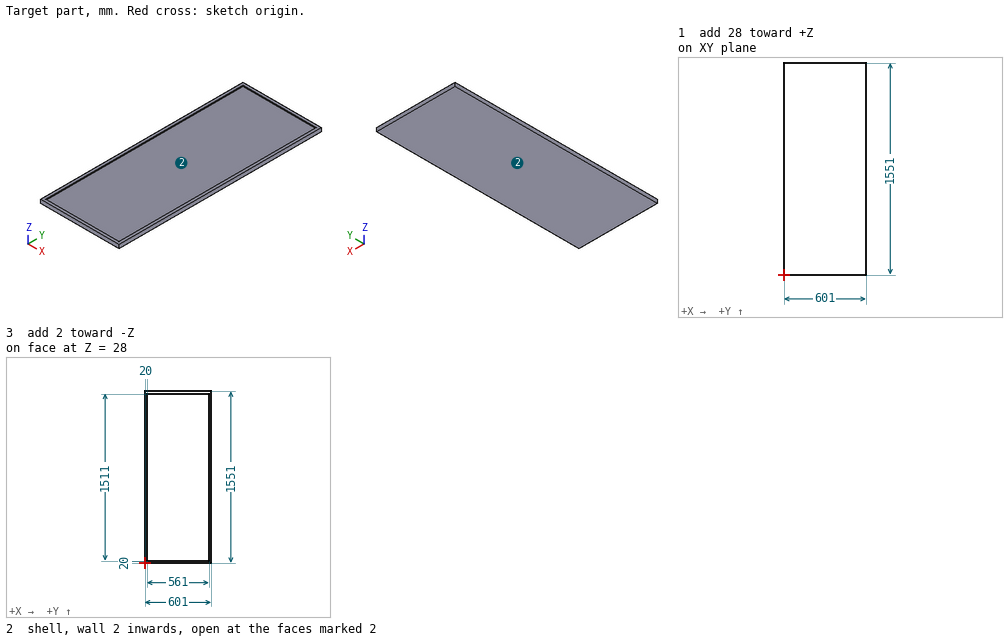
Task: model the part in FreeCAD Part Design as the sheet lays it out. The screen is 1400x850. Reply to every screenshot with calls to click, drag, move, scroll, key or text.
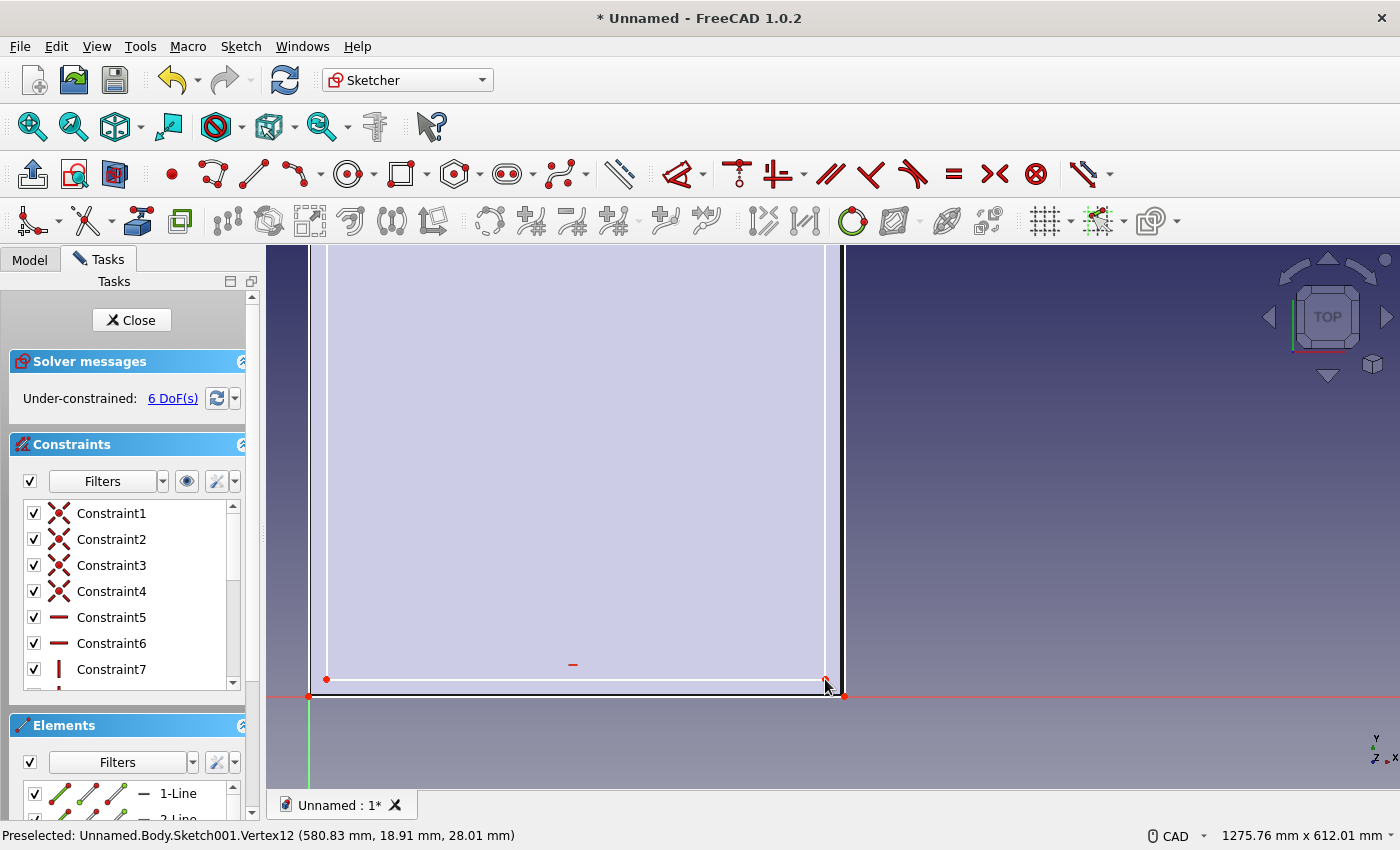
click(676, 174)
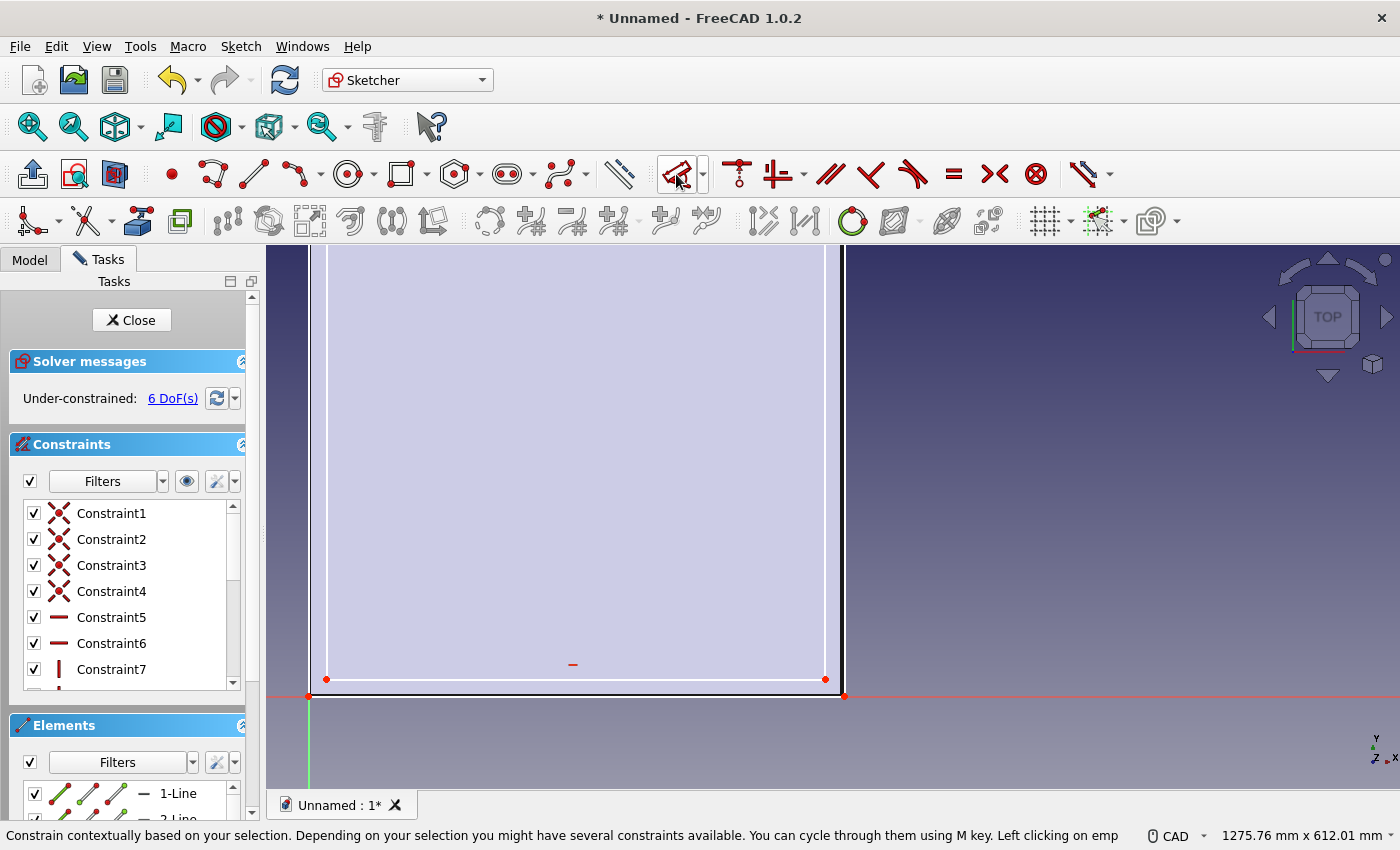
click(470, 697)
click(577, 731)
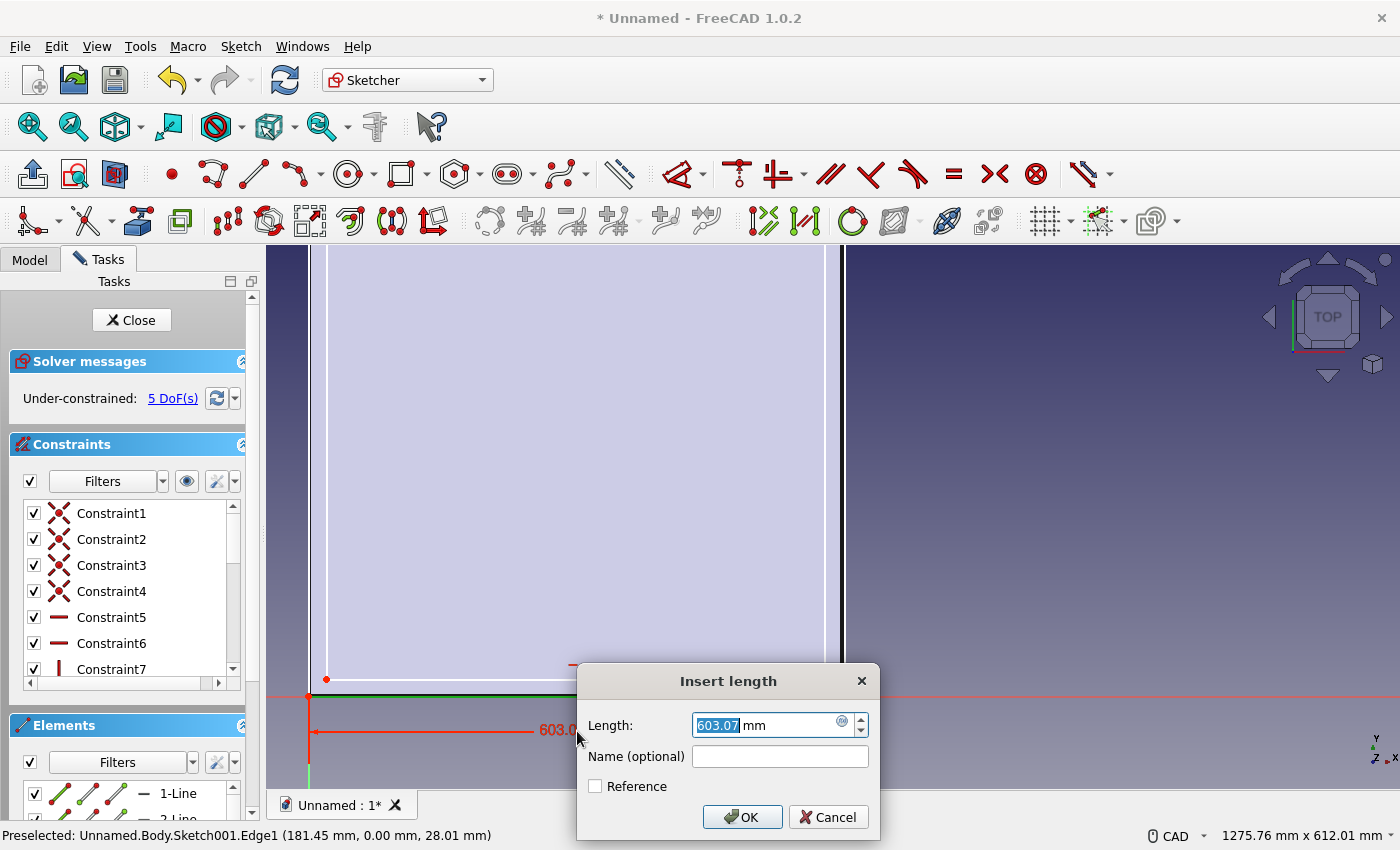
text(601)
key(Return)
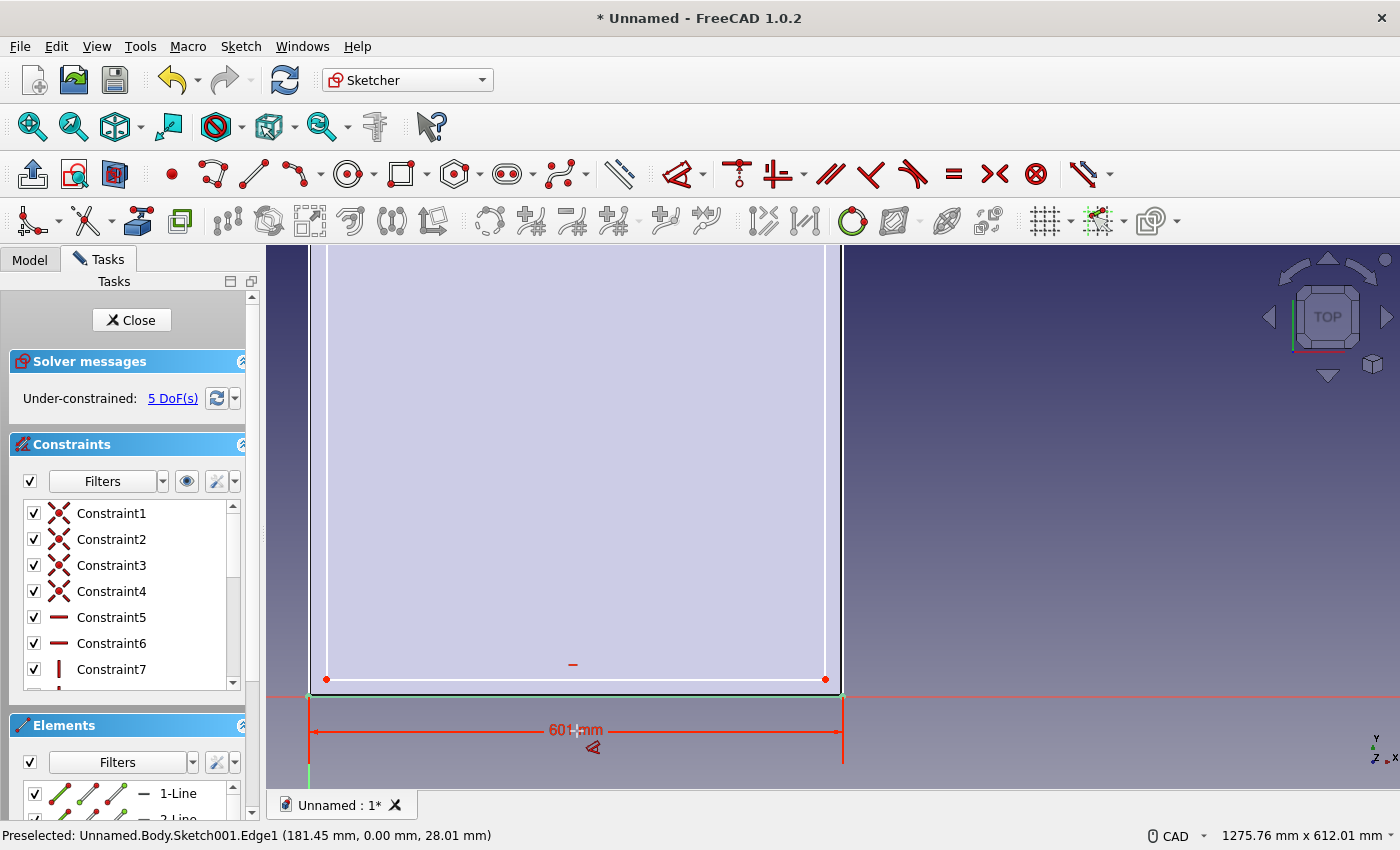
click(476, 680)
click(461, 714)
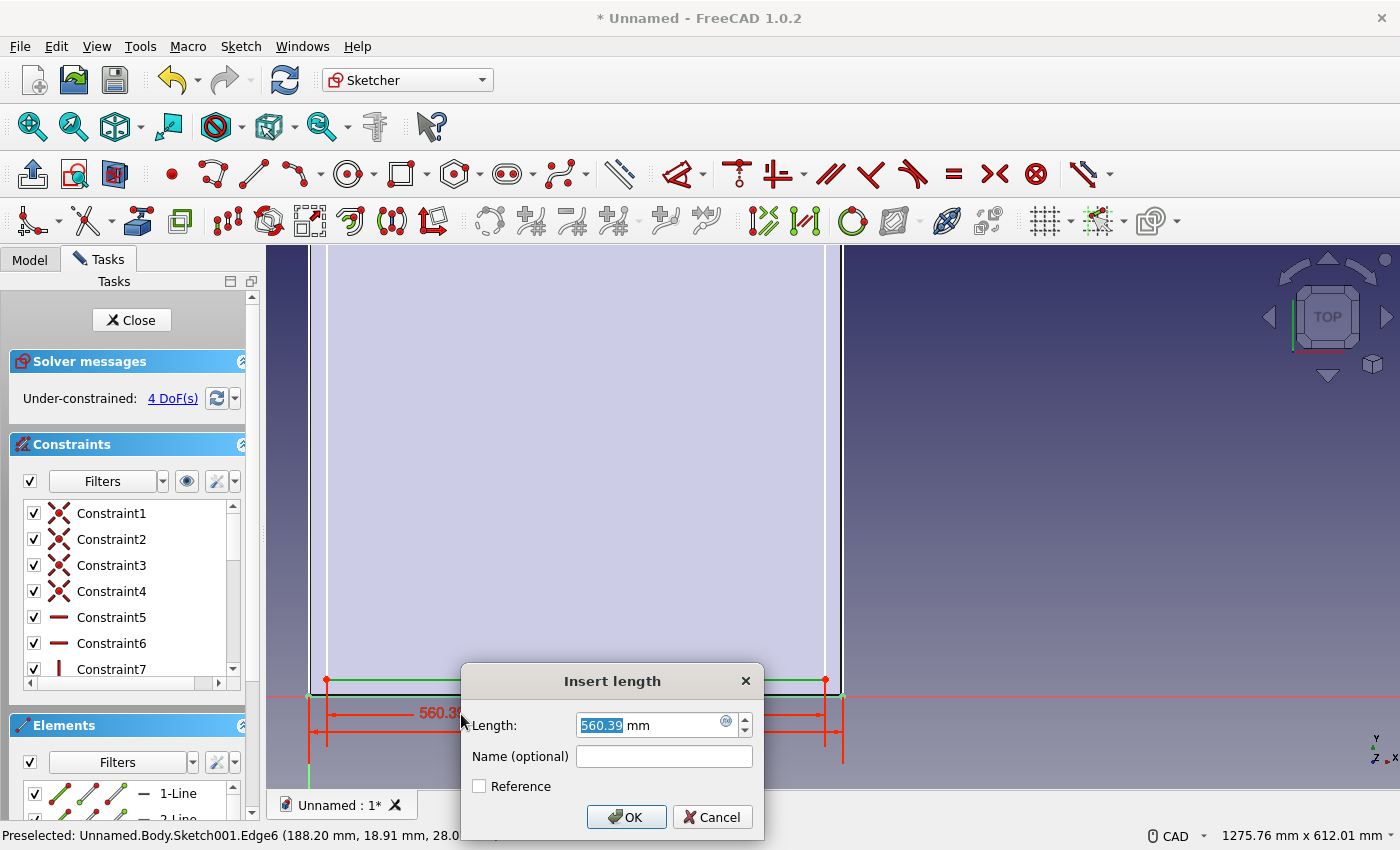
text(561)
key(Return)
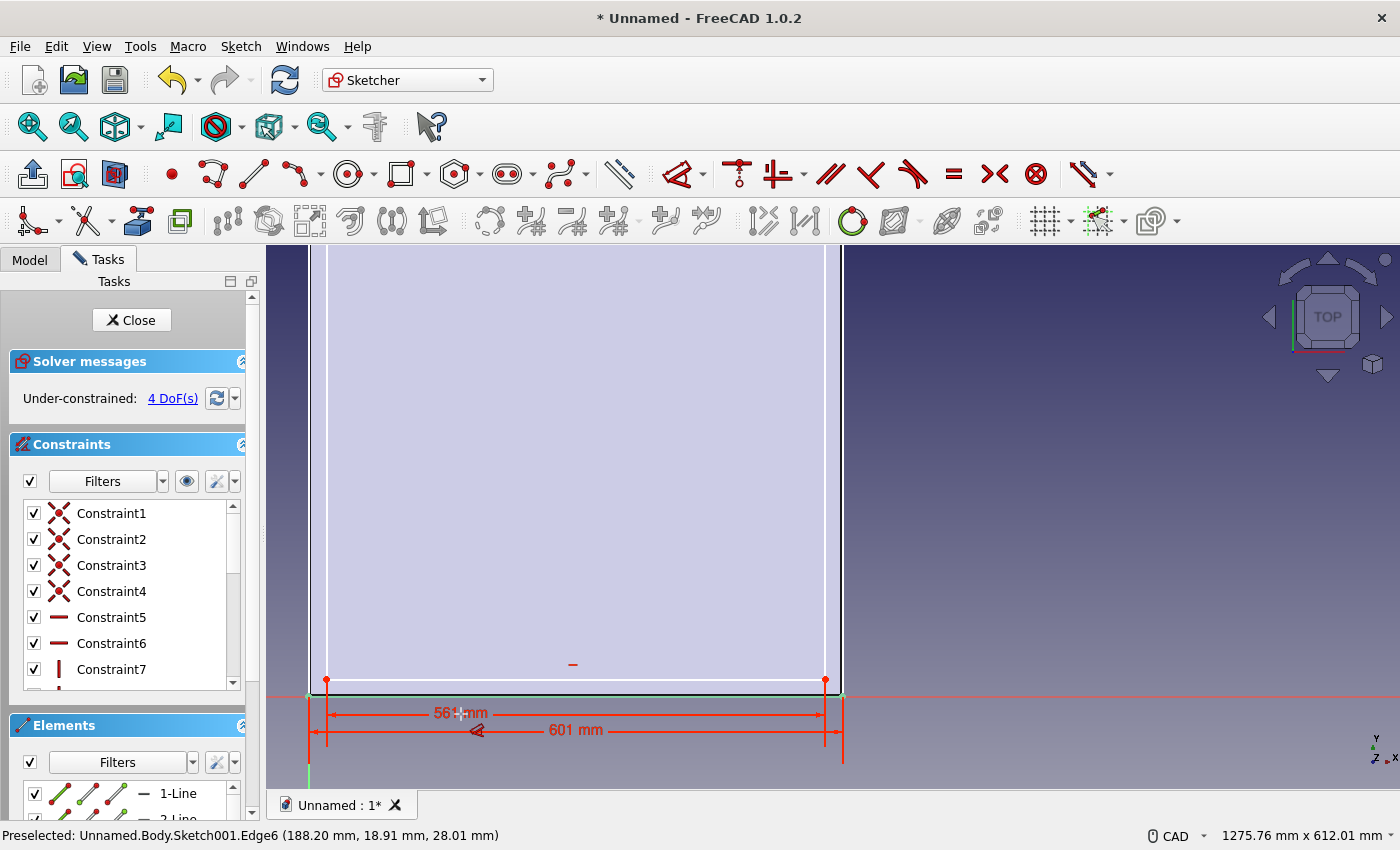
scroll(826, 684, down, 7)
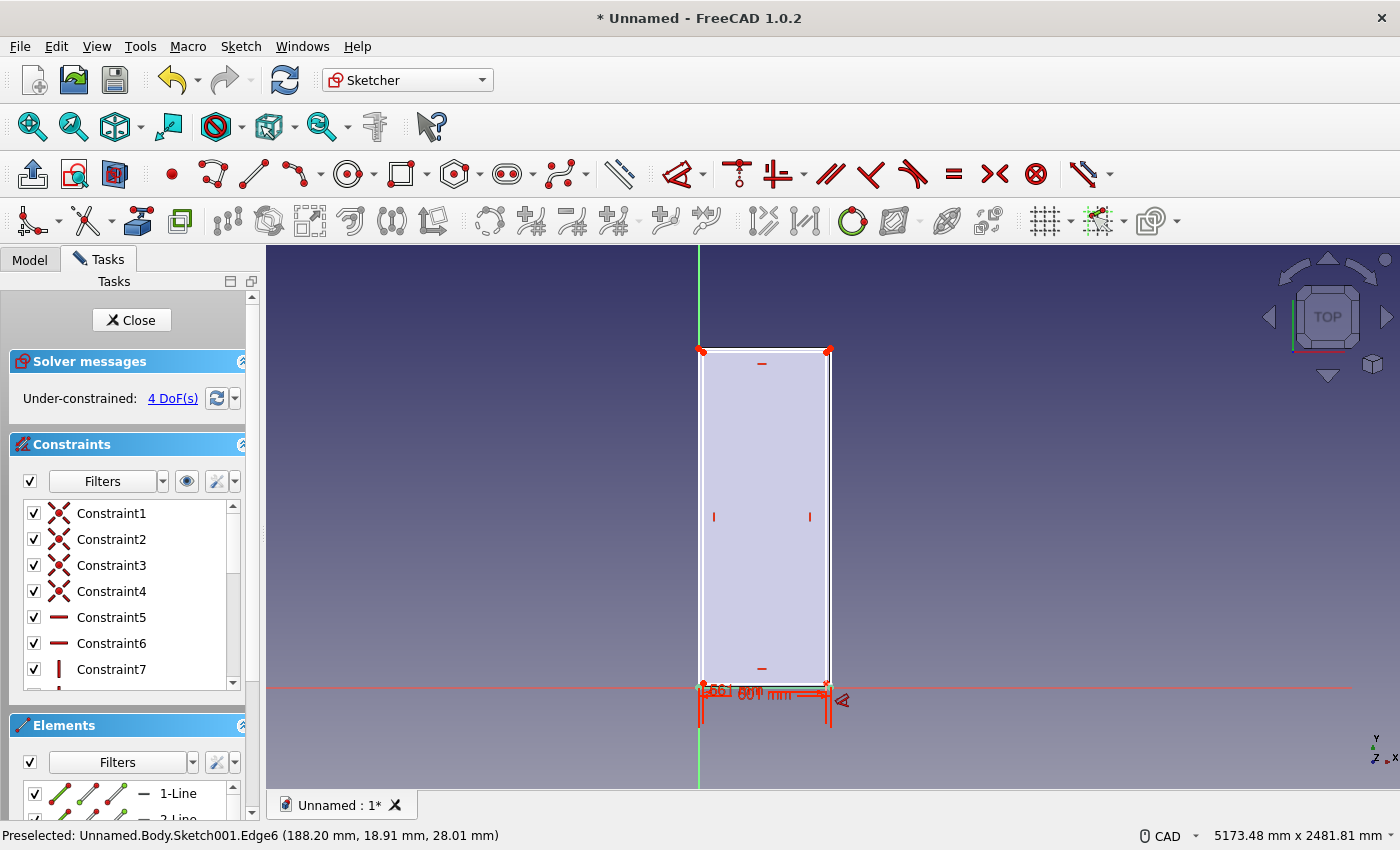
scroll(703, 352, up, 12)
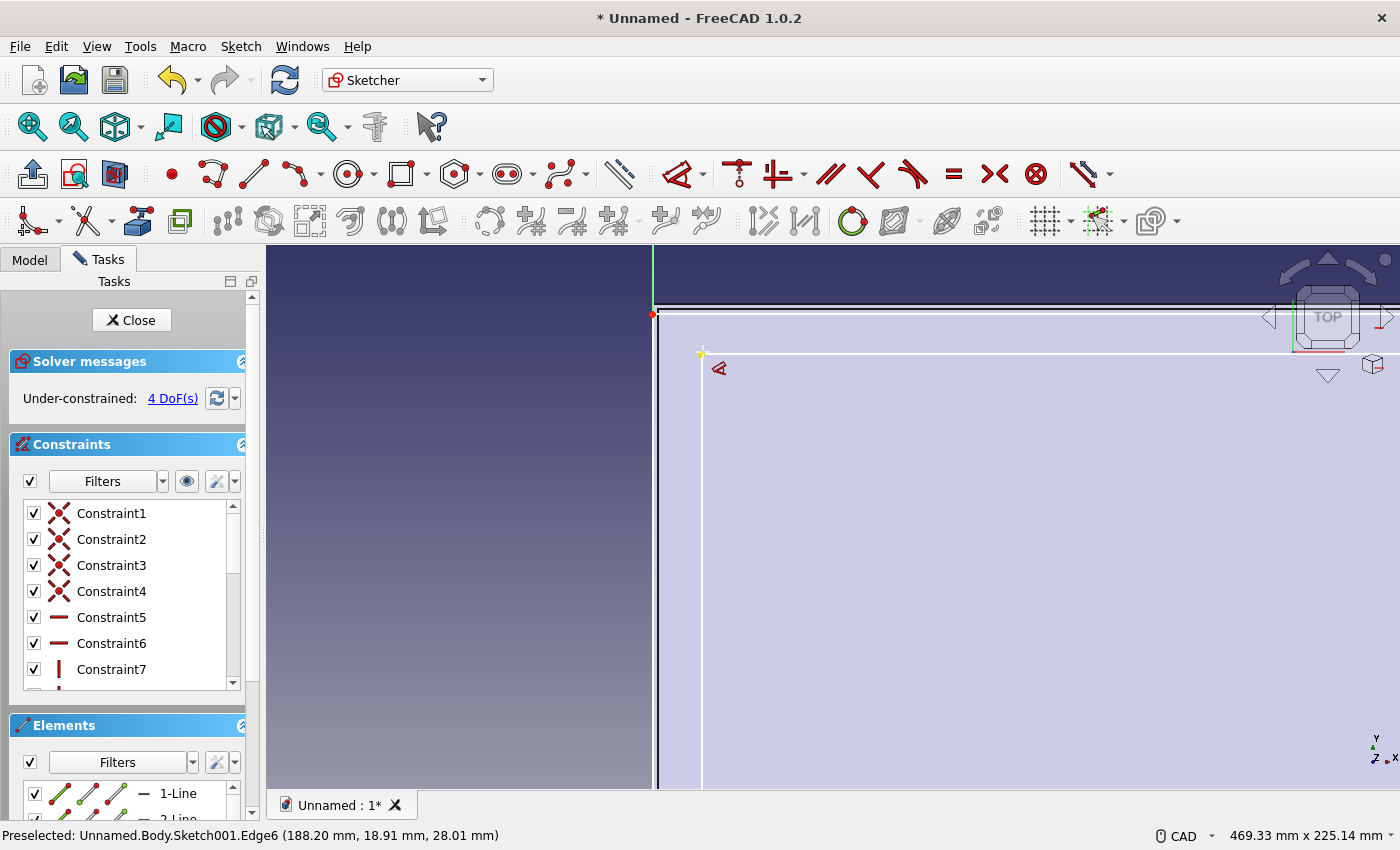
click(702, 354)
click(677, 296)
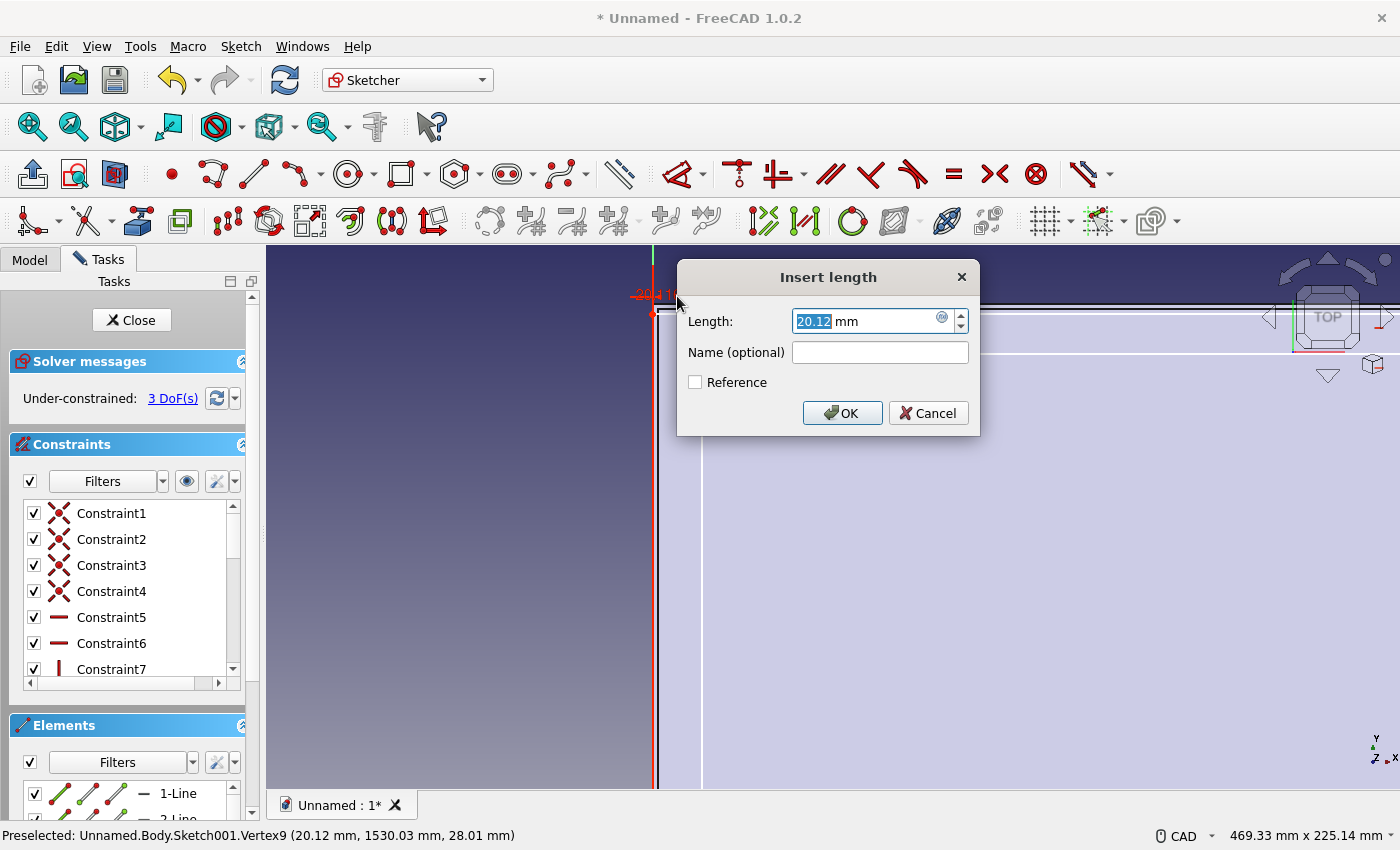
text(20)
key(Return)